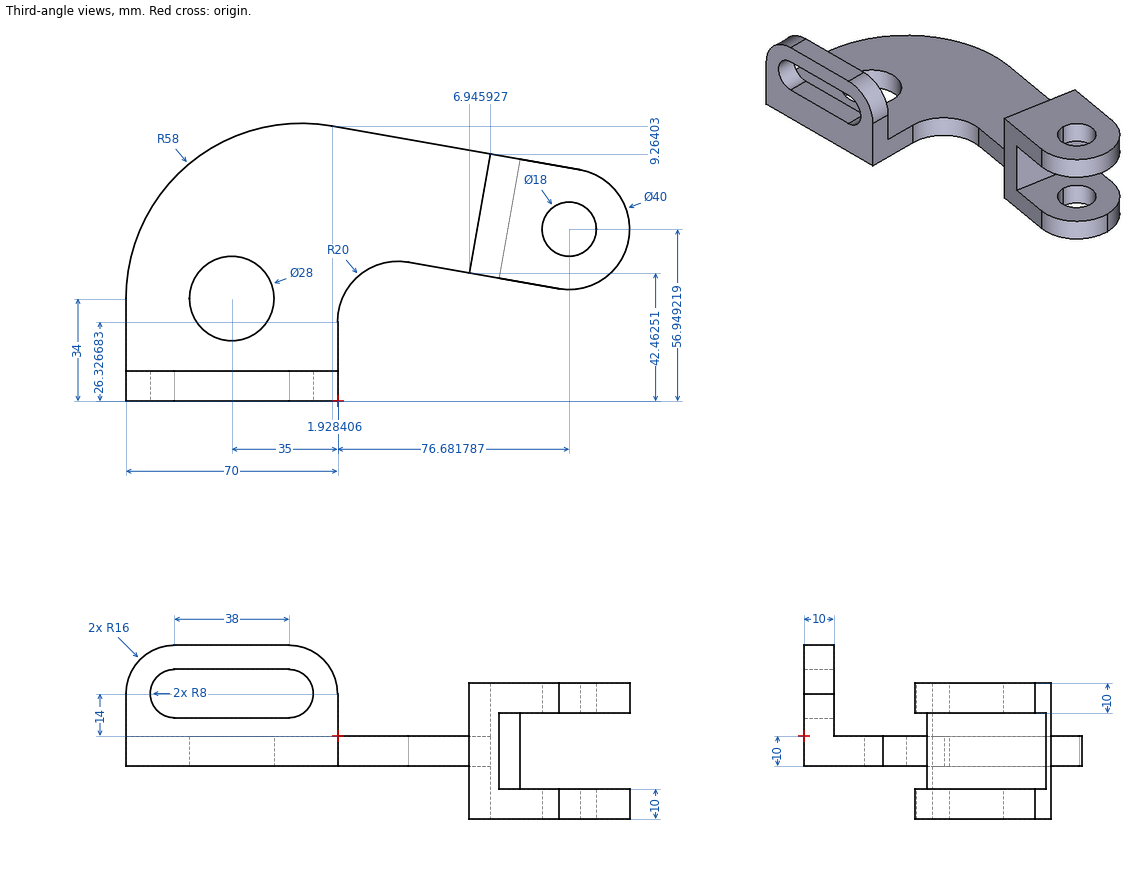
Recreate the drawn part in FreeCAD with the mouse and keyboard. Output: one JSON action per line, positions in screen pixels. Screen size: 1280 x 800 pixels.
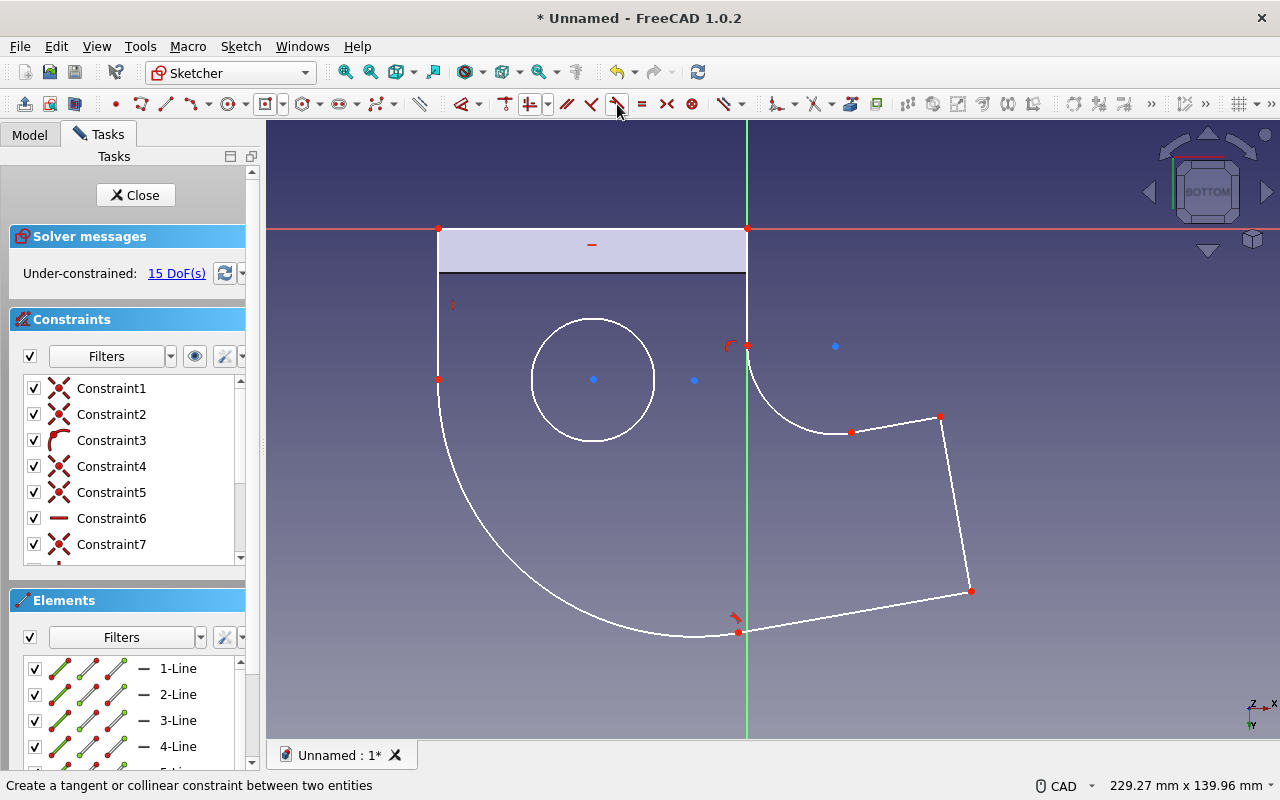
{"action": "left_click", "coordinate": [913, 422]}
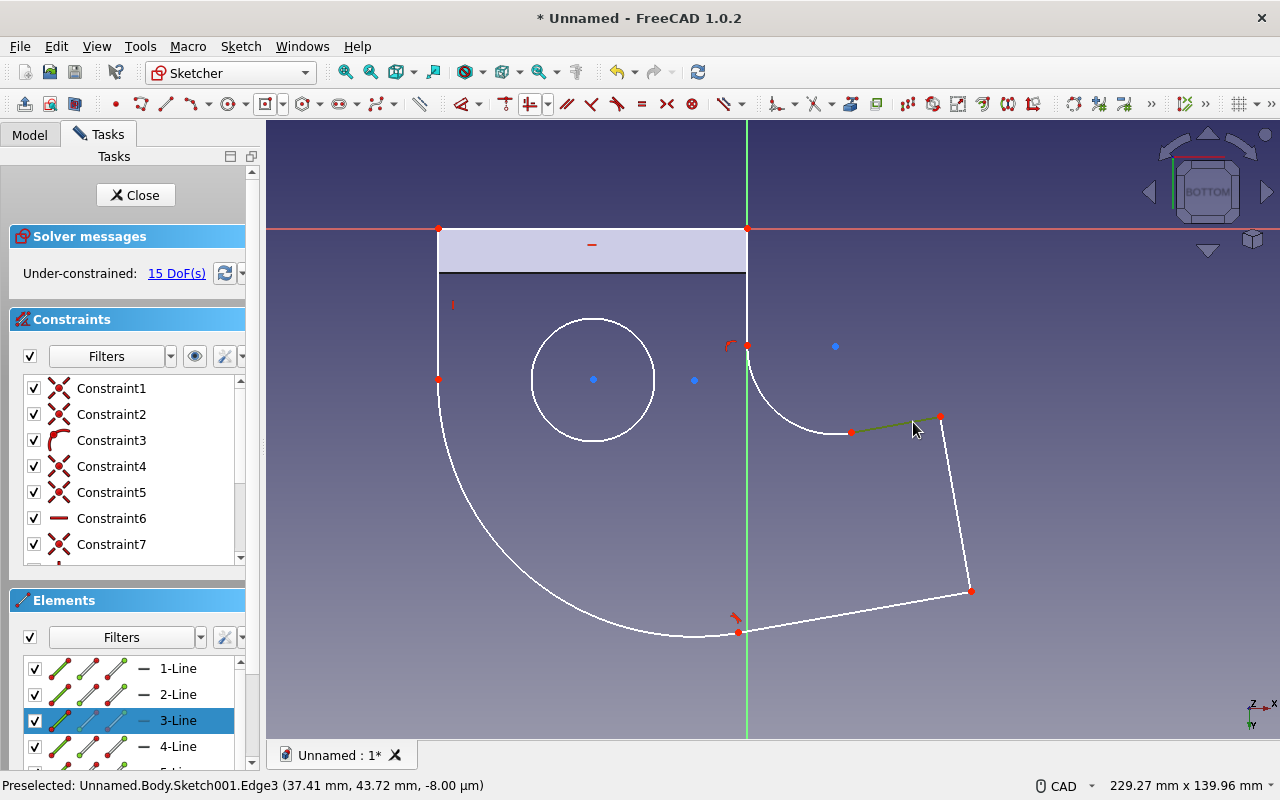
{"action": "left_click", "coordinate": [759, 390]}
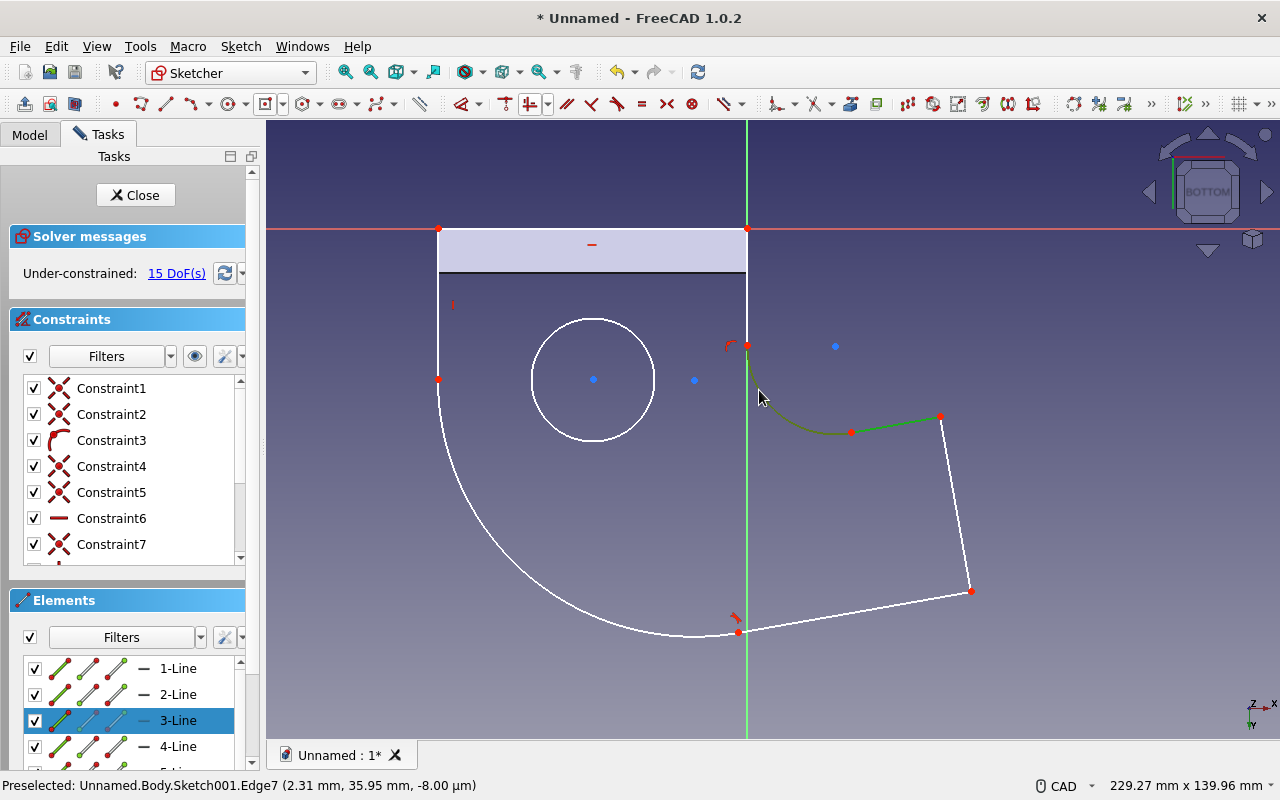
{"action": "left_click", "coordinate": [617, 104]}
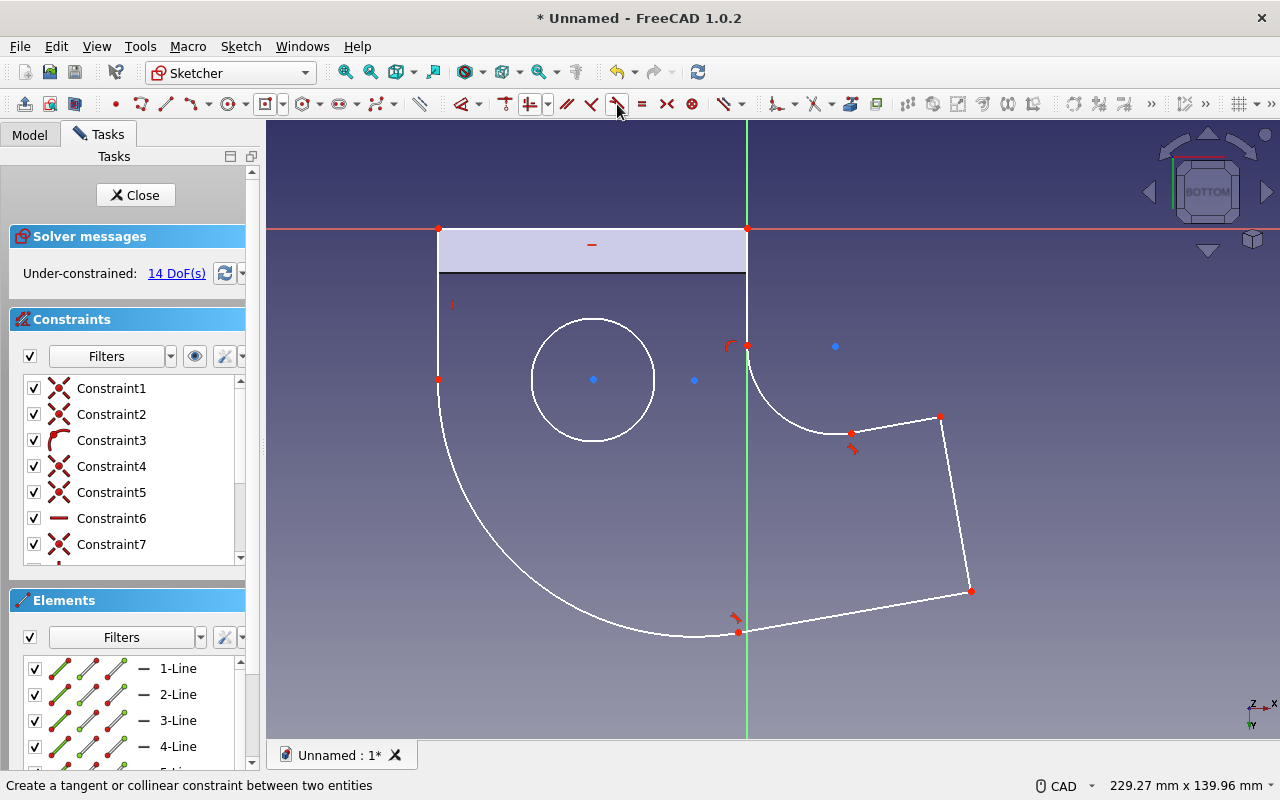
{"action": "left_click", "coordinate": [747, 311]}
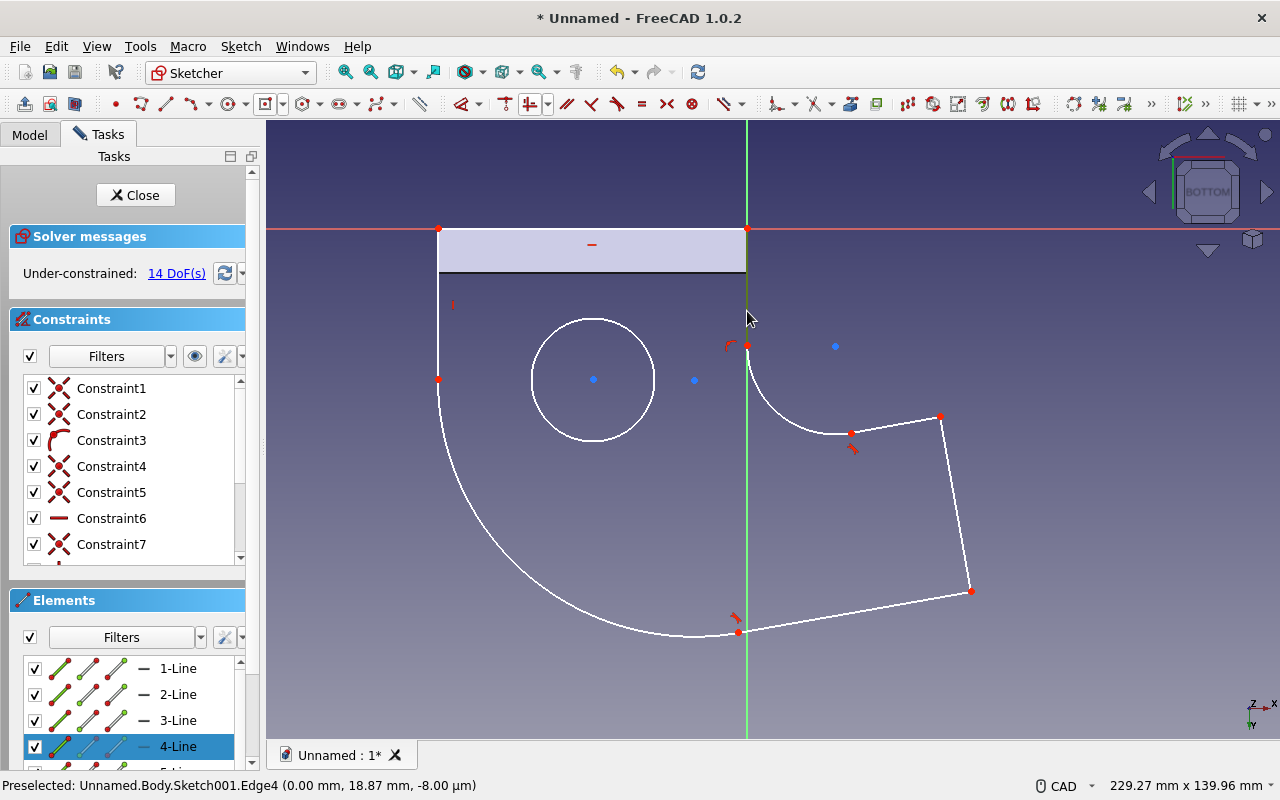
{"action": "left_click", "coordinate": [759, 390]}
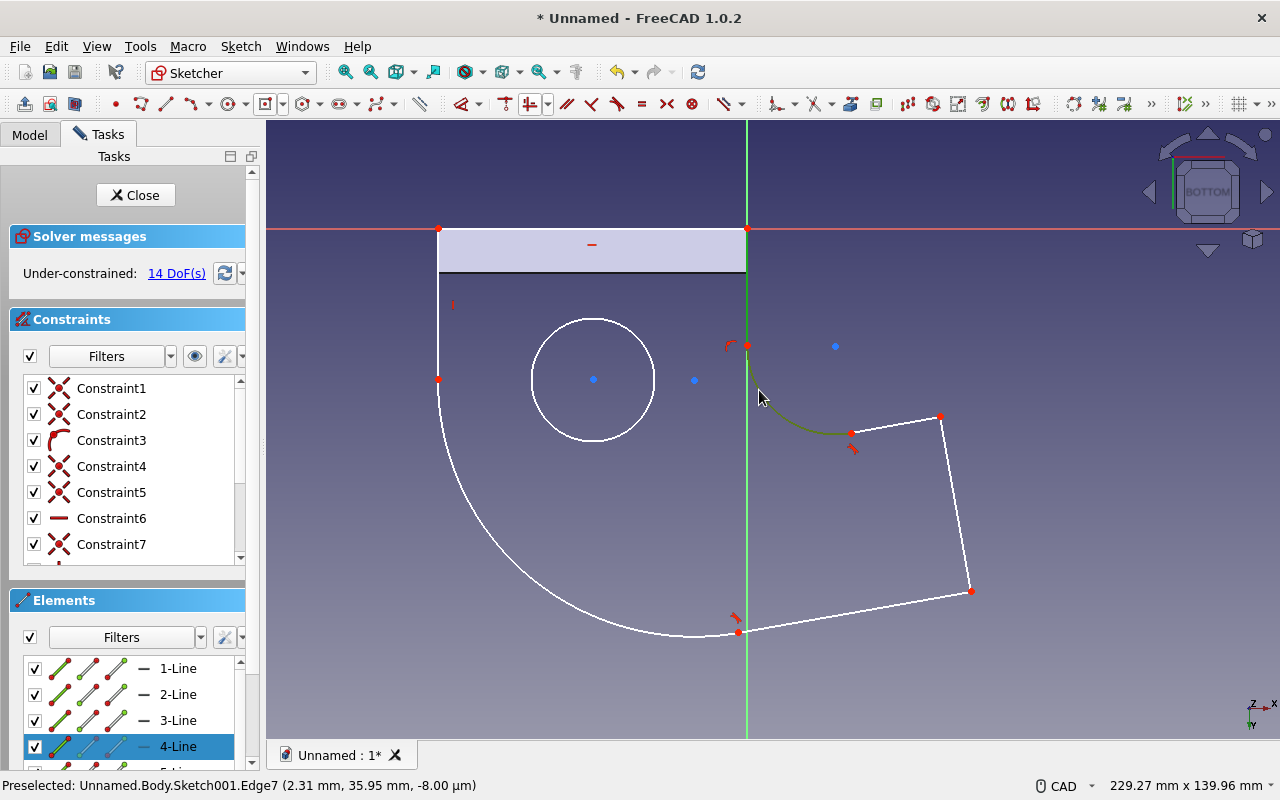
{"action": "left_click", "coordinate": [617, 104]}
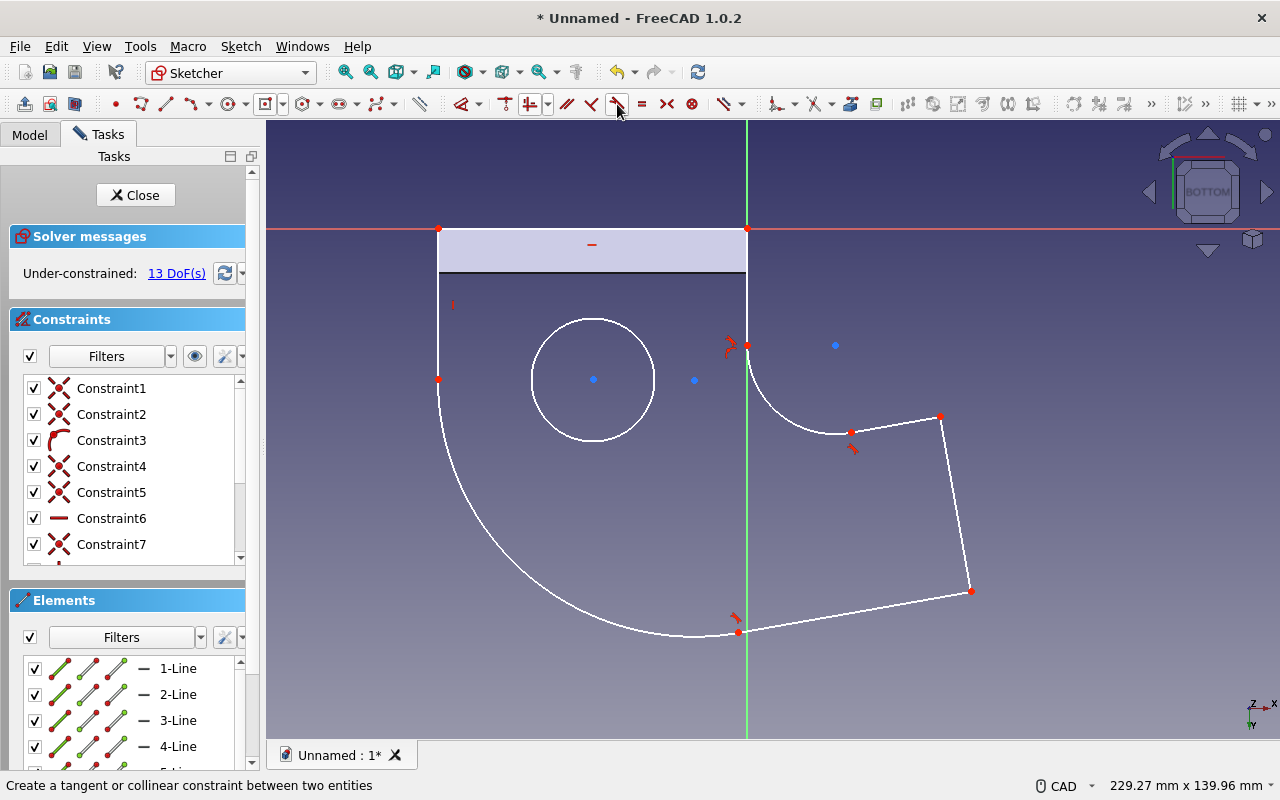
{"action": "left_click", "coordinate": [460, 104]}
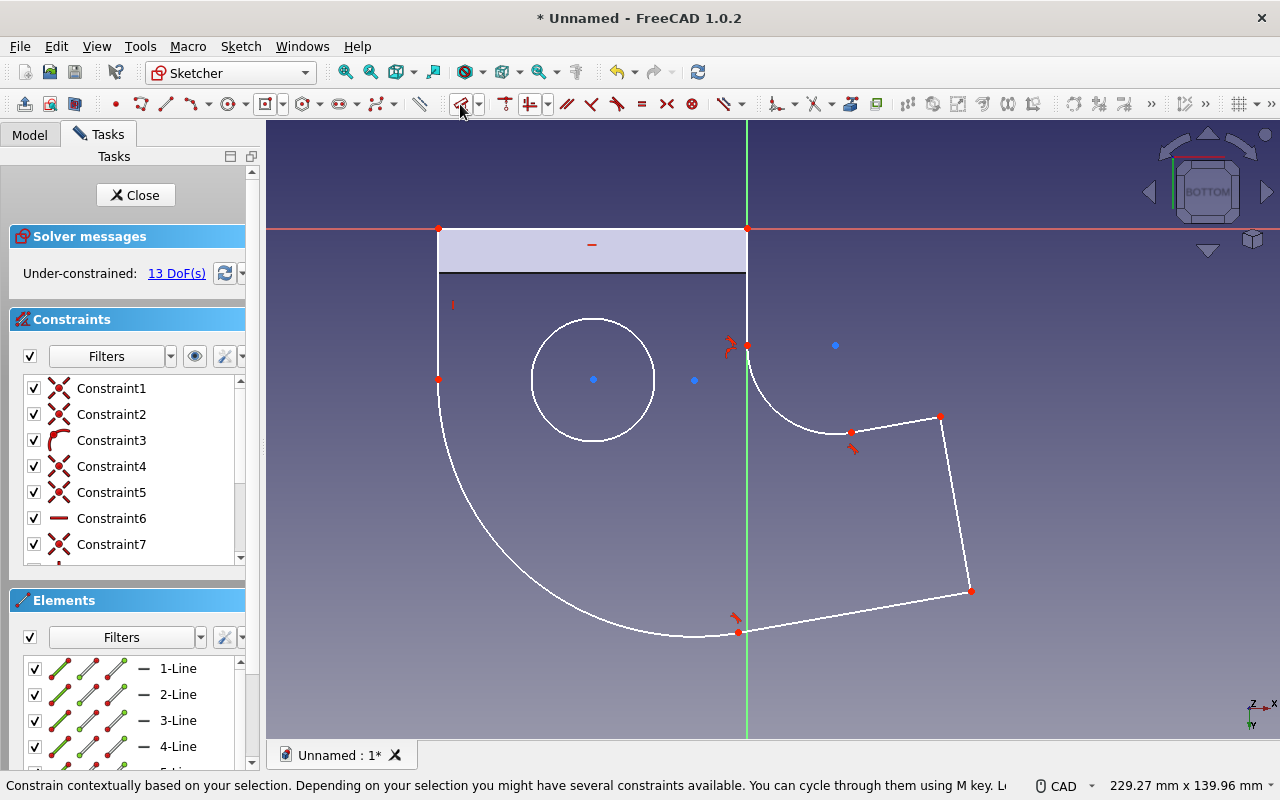
{"action": "left_click", "coordinate": [759, 390]}
{"action": "left_click", "coordinate": [731, 406]}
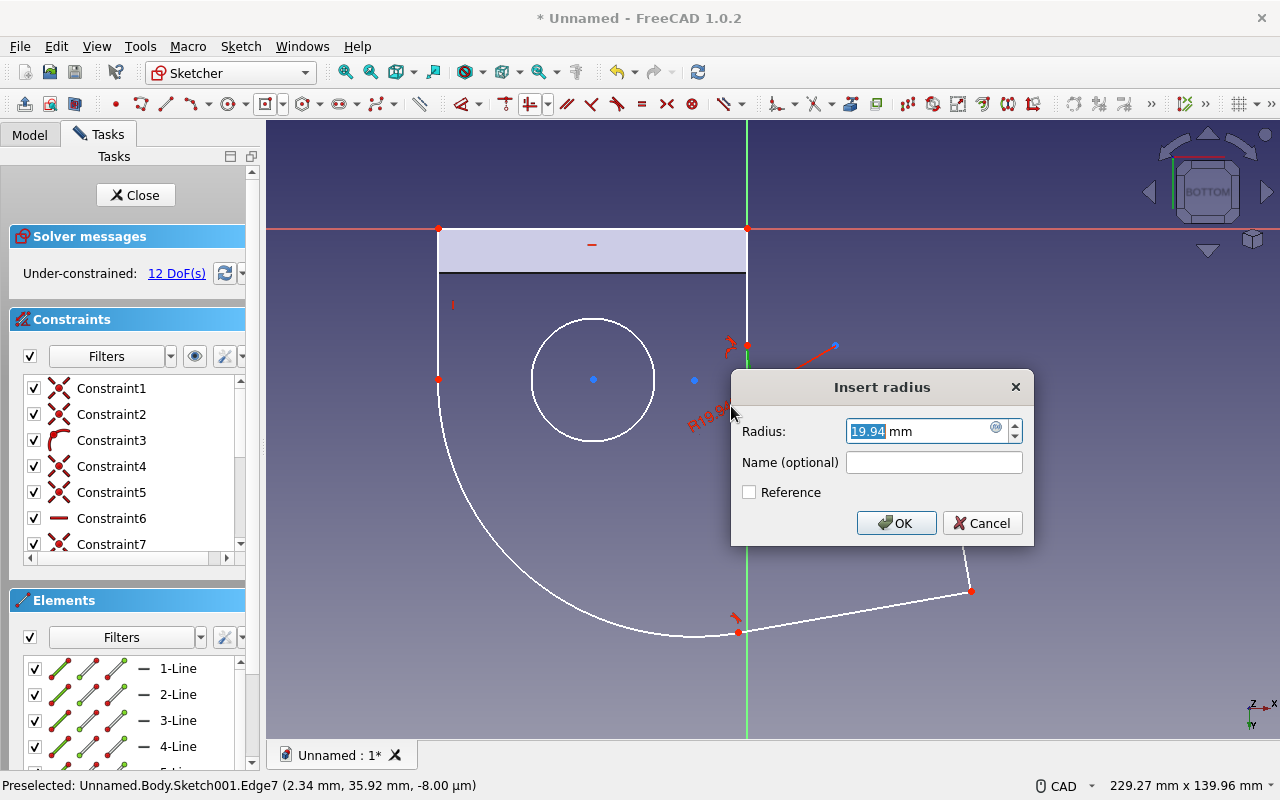
{"action": "type", "text": "20"}
{"action": "key", "text": "Return"}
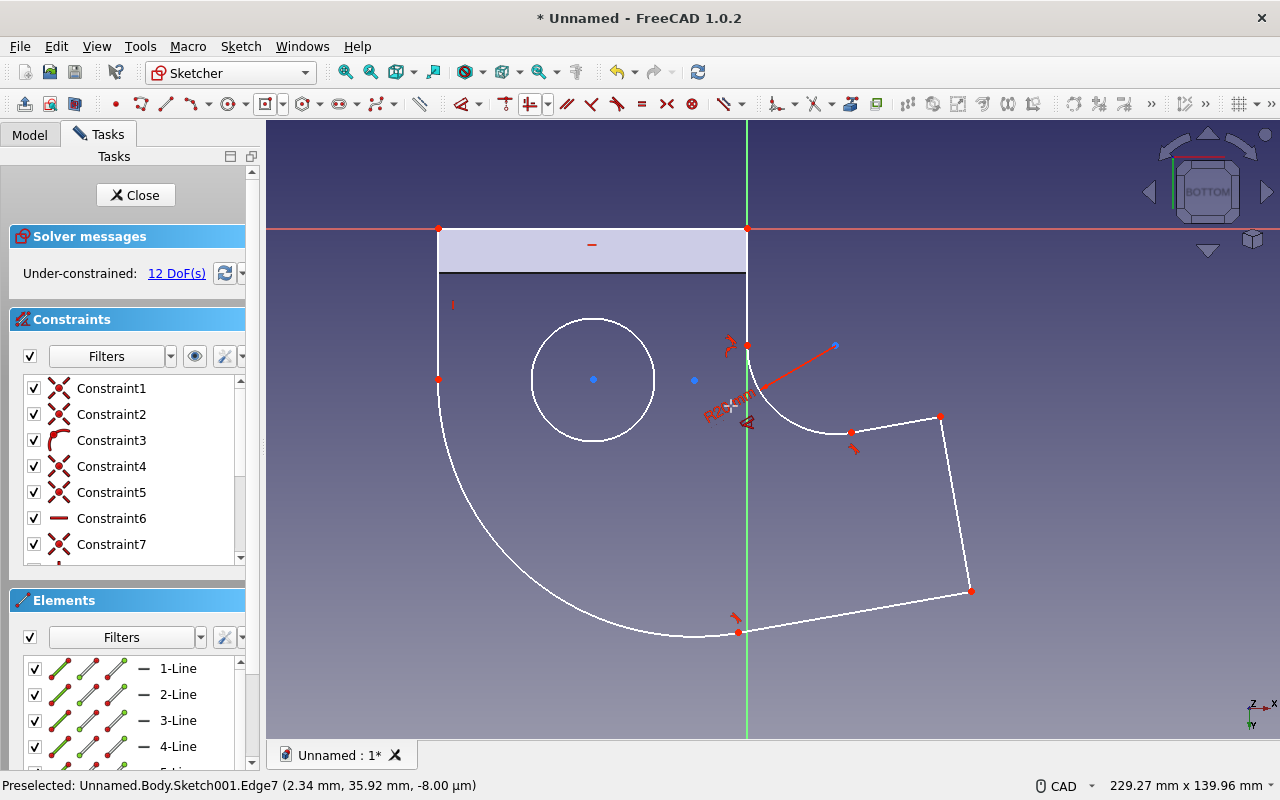
{"action": "left_click", "coordinate": [472, 508]}
{"action": "left_click", "coordinate": [444, 524]}